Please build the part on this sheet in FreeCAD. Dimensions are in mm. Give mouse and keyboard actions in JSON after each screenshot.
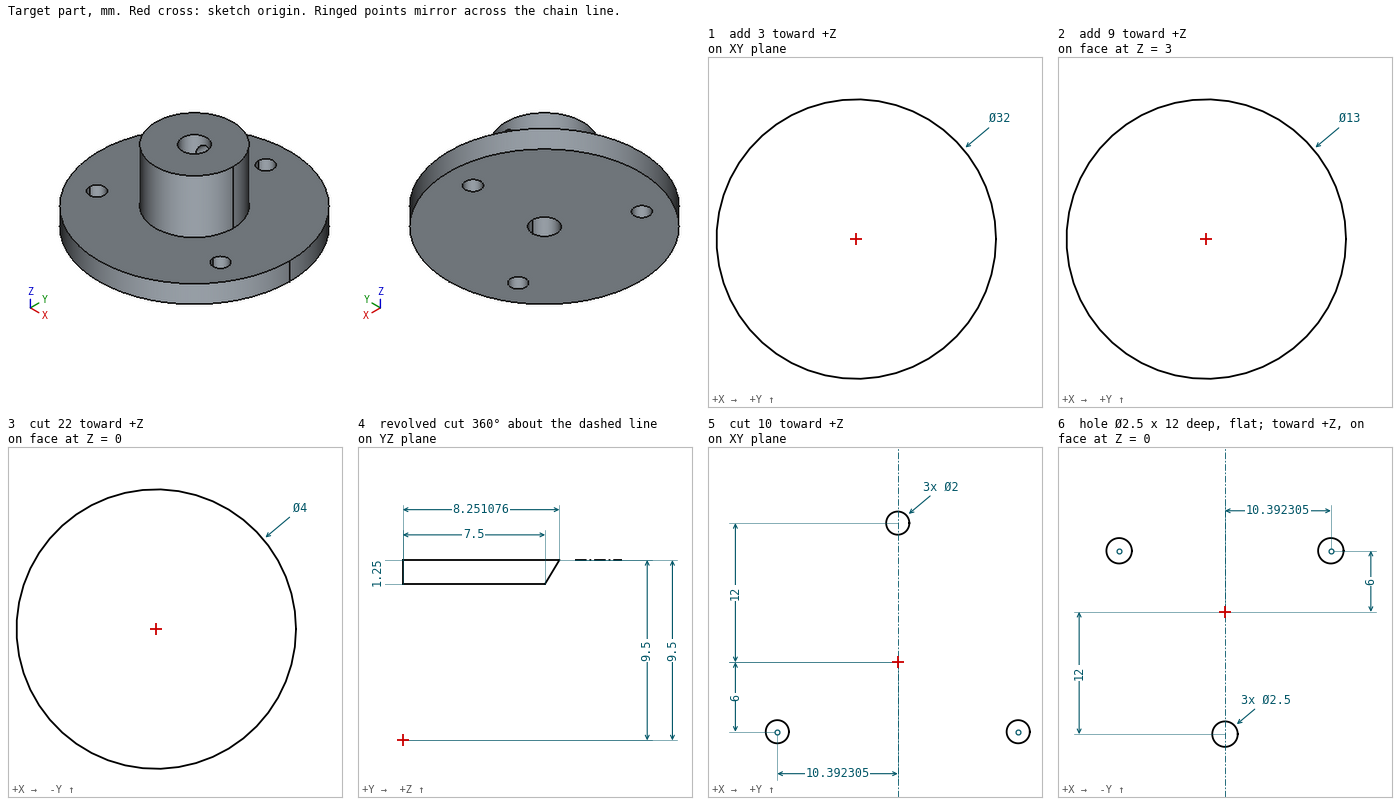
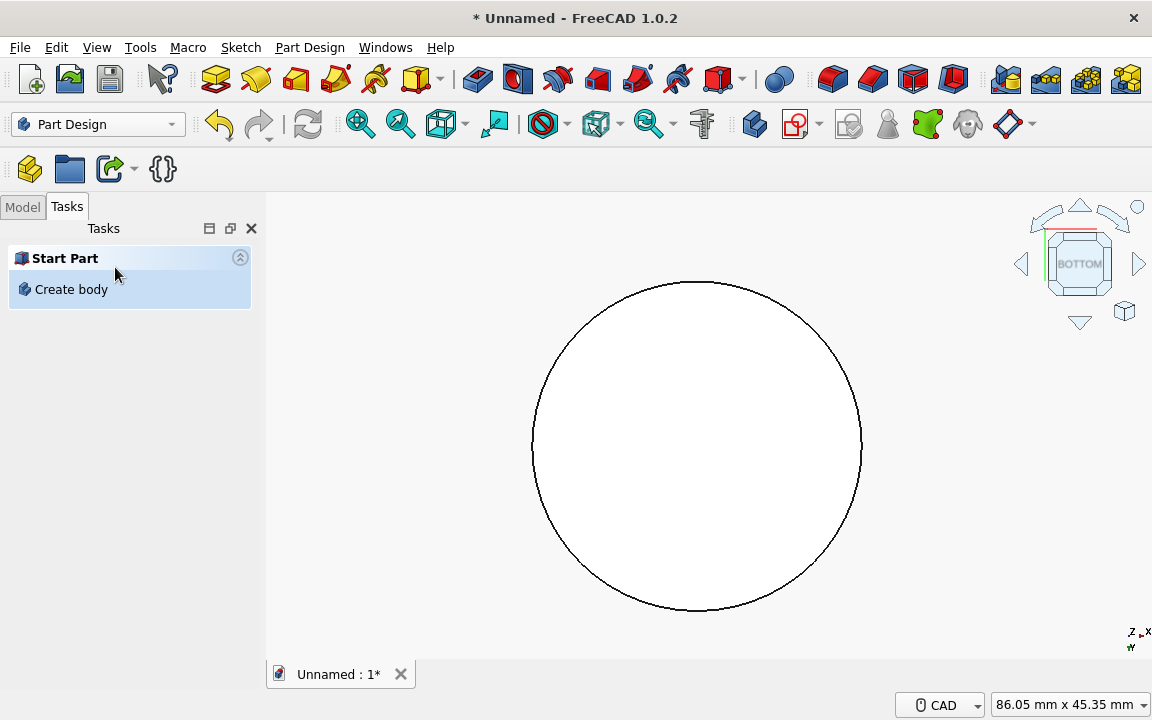
{"action": "left_click", "coordinate": [697, 445]}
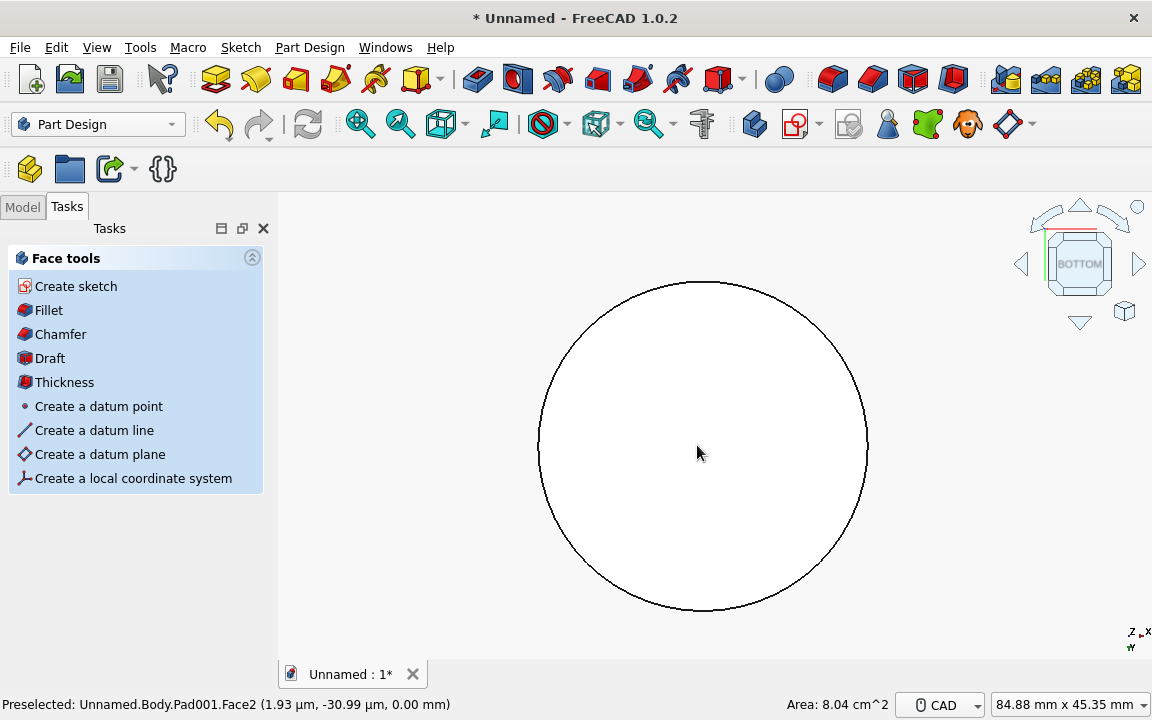
{"action": "left_click", "coordinate": [796, 124]}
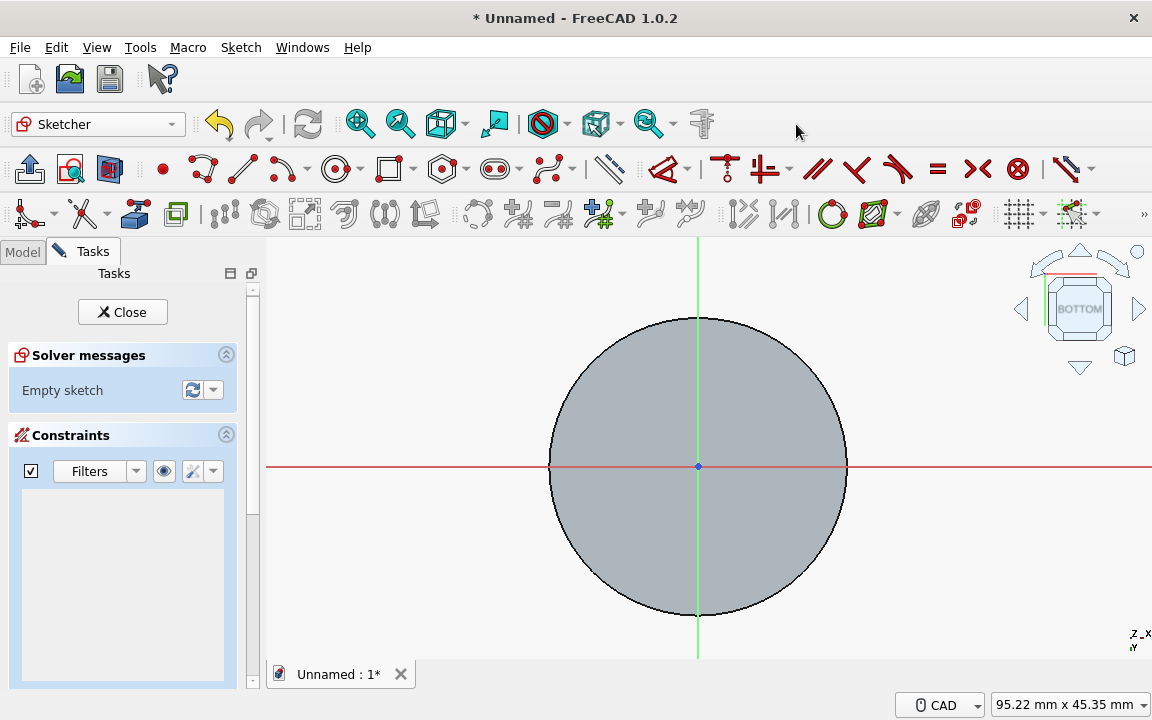
{"action": "scroll", "coordinate": [707, 470], "scroll_direction": "up", "scroll_amount": 10}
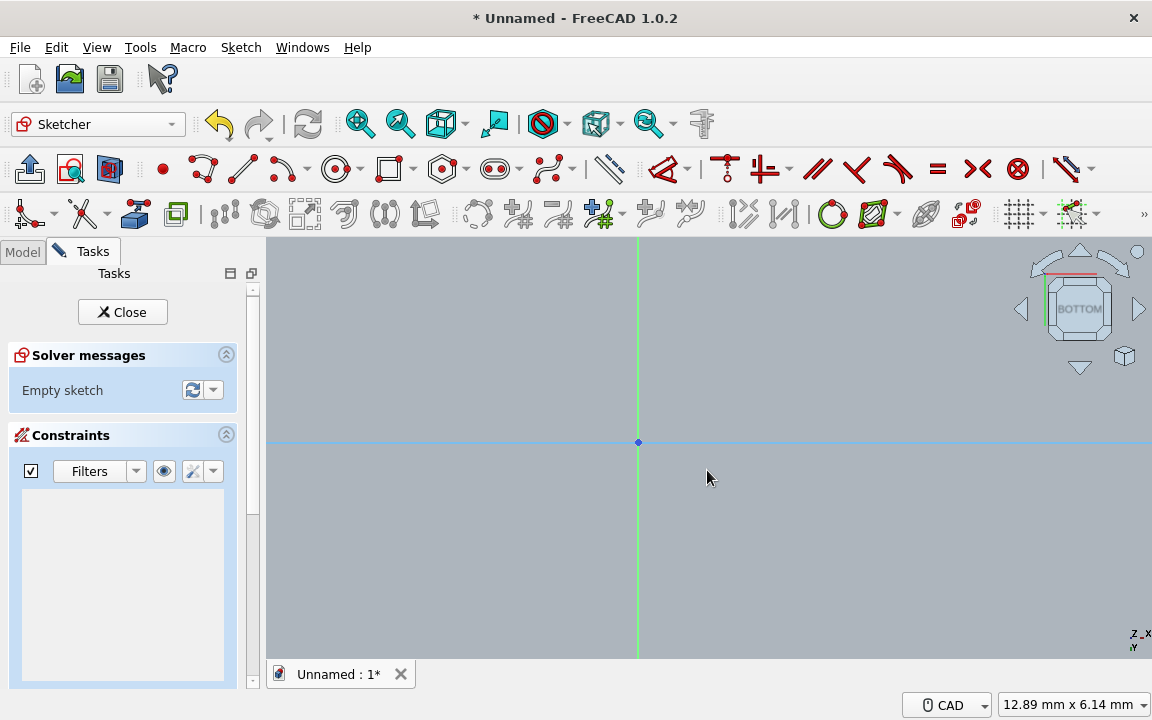
{"action": "left_click", "coordinate": [336, 170]}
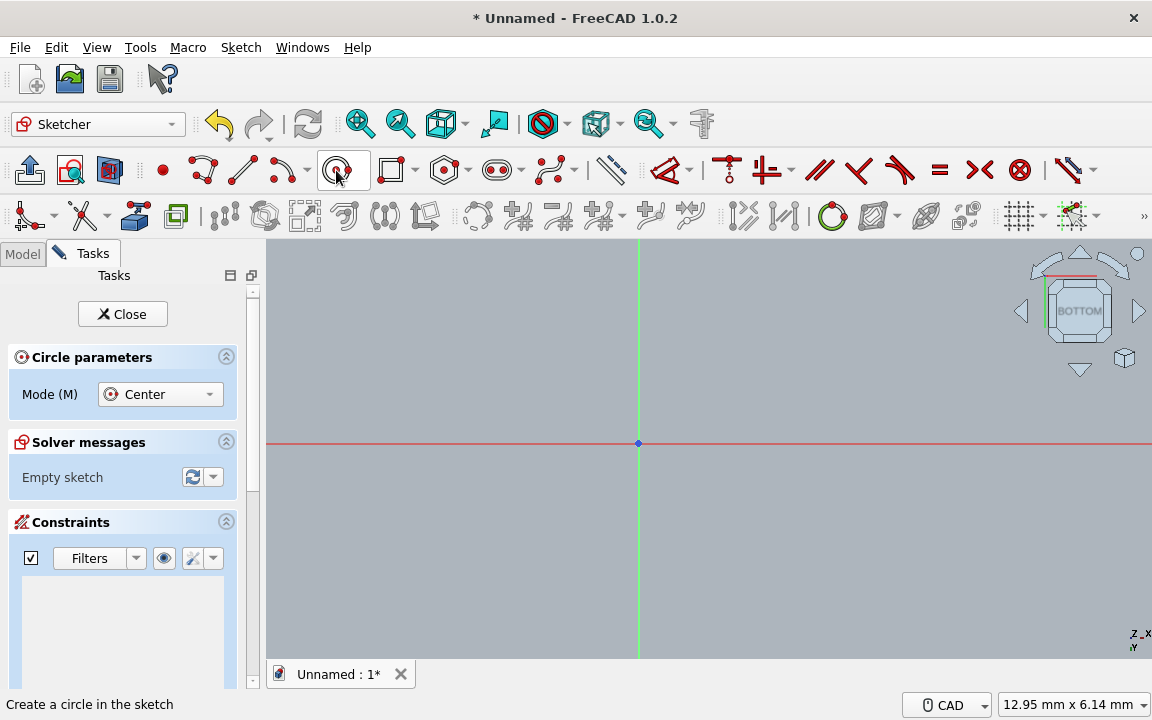
{"action": "left_click", "coordinate": [639, 444]}
{"action": "mouse_move", "coordinate": [735, 347]}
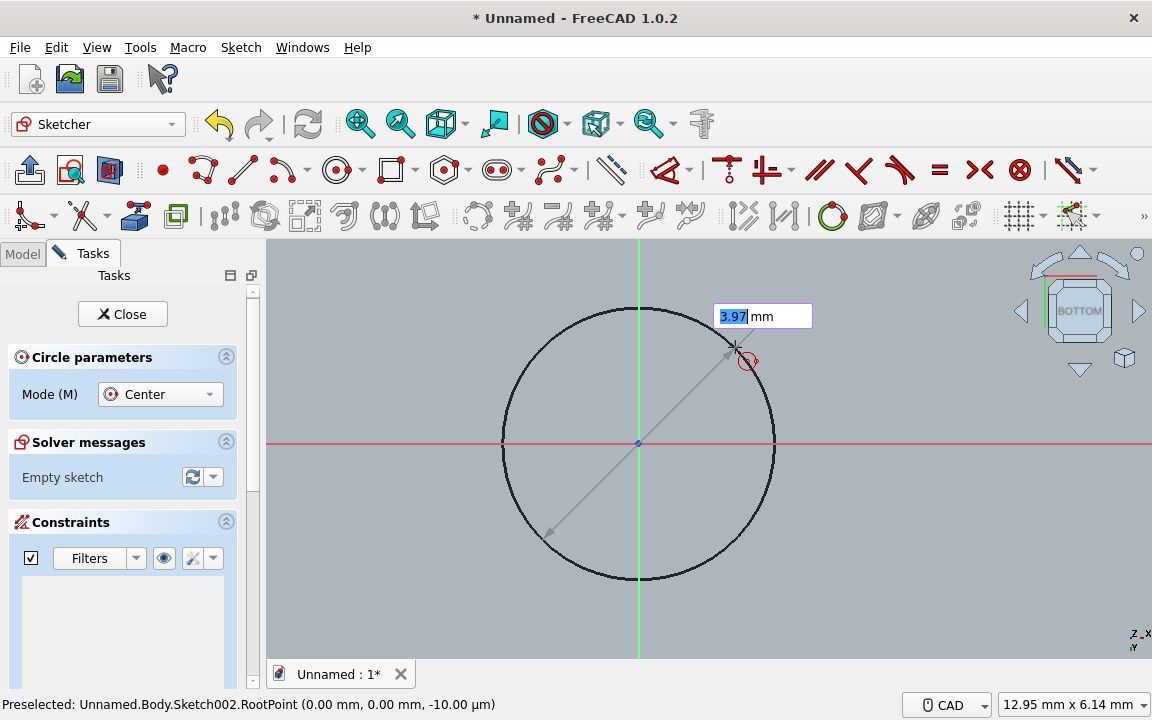
{"action": "type", "text": "4"}
{"action": "key", "text": "Return"}
{"action": "key", "text": "Escape"}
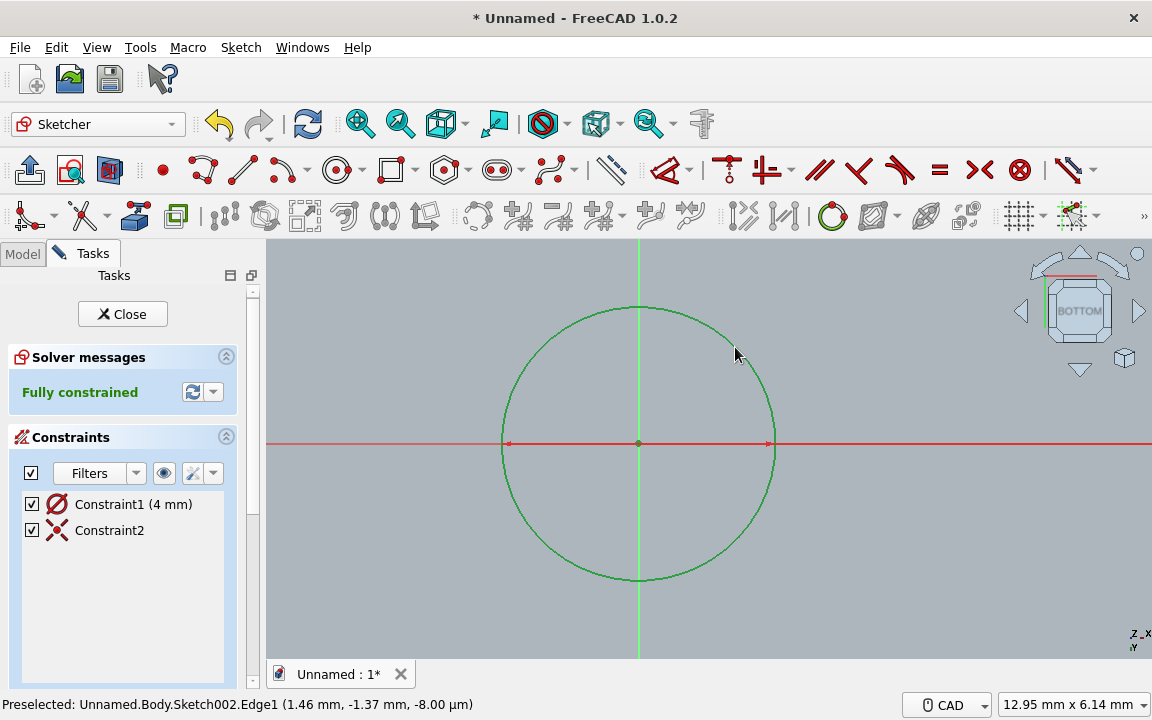
{"action": "left_click", "coordinate": [123, 314]}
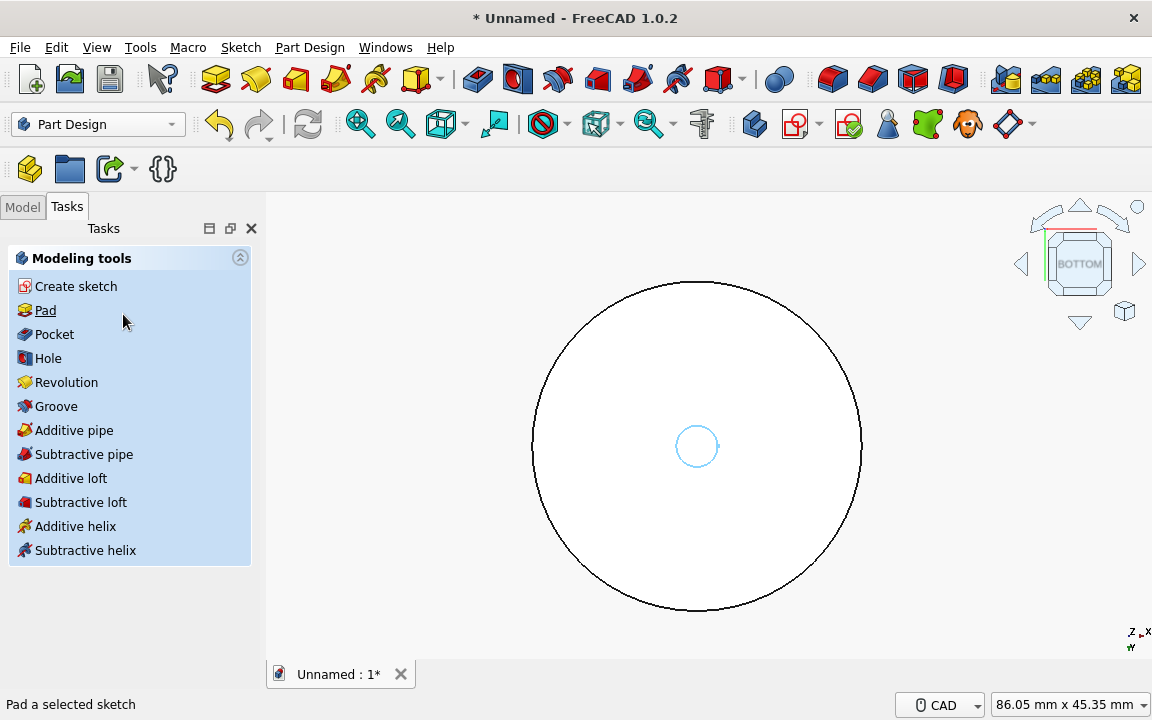
{"action": "left_click", "coordinate": [478, 80]}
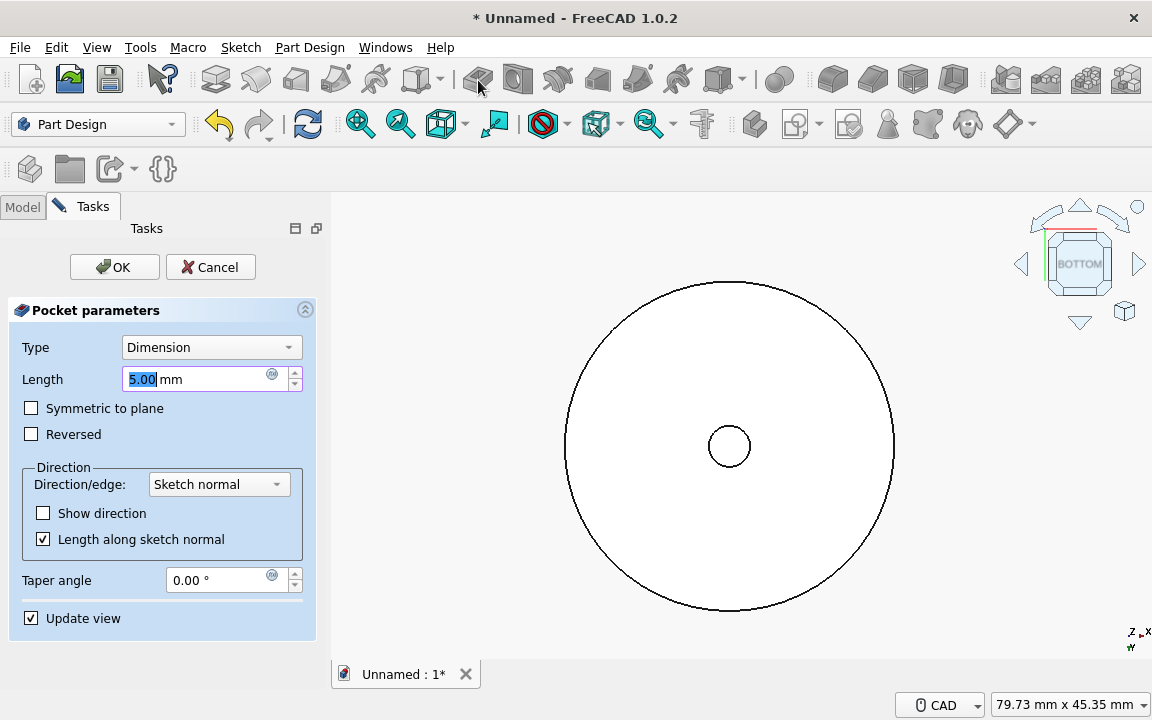
{"action": "type", "text": "22"}
{"action": "key", "text": "Tab"}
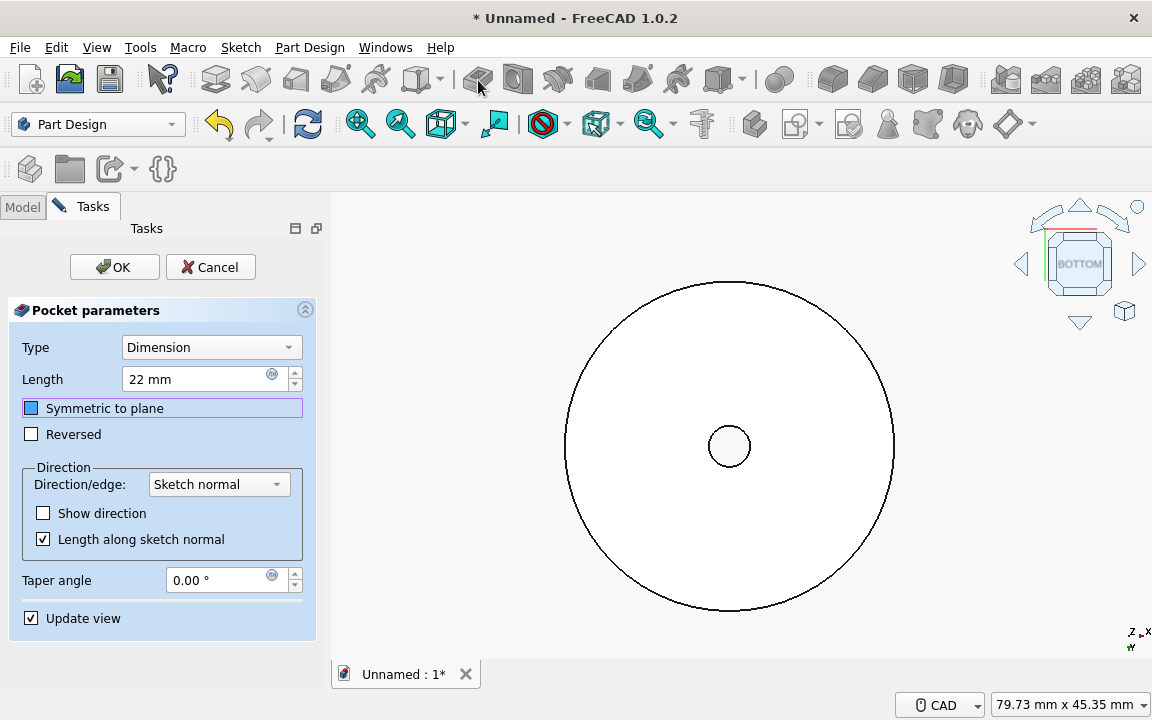
{"action": "left_click", "coordinate": [115, 267]}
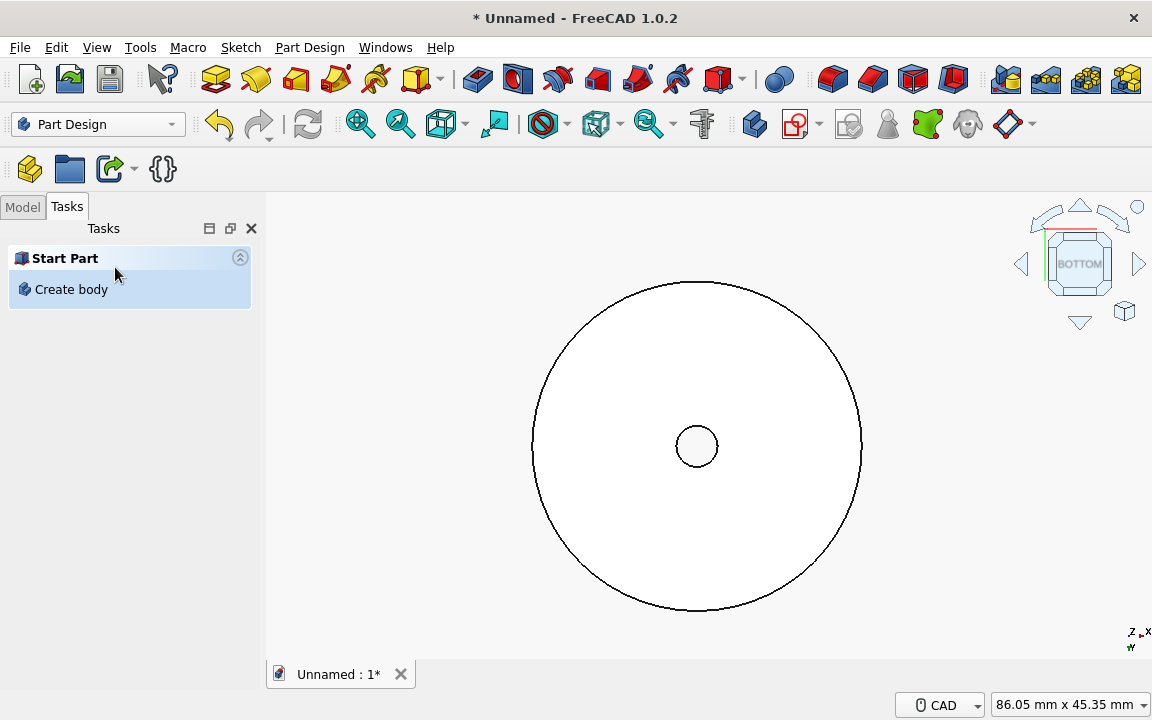
{"action": "left_click", "coordinate": [796, 124]}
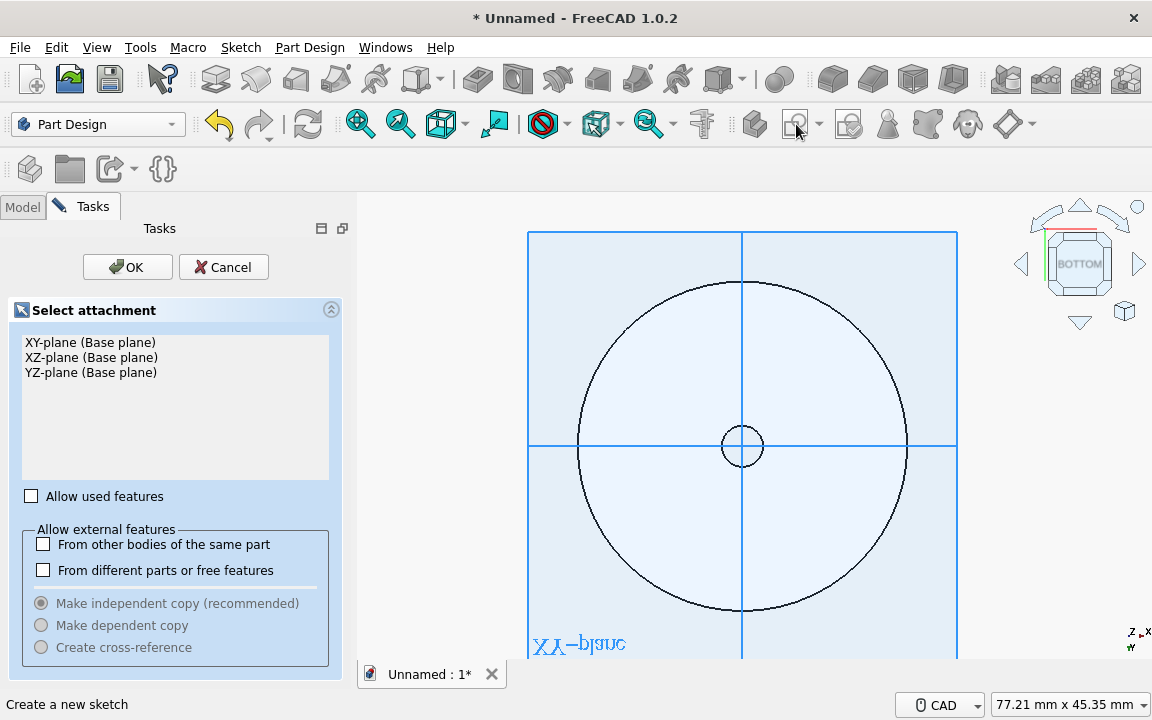
{"action": "left_click", "coordinate": [82, 372]}